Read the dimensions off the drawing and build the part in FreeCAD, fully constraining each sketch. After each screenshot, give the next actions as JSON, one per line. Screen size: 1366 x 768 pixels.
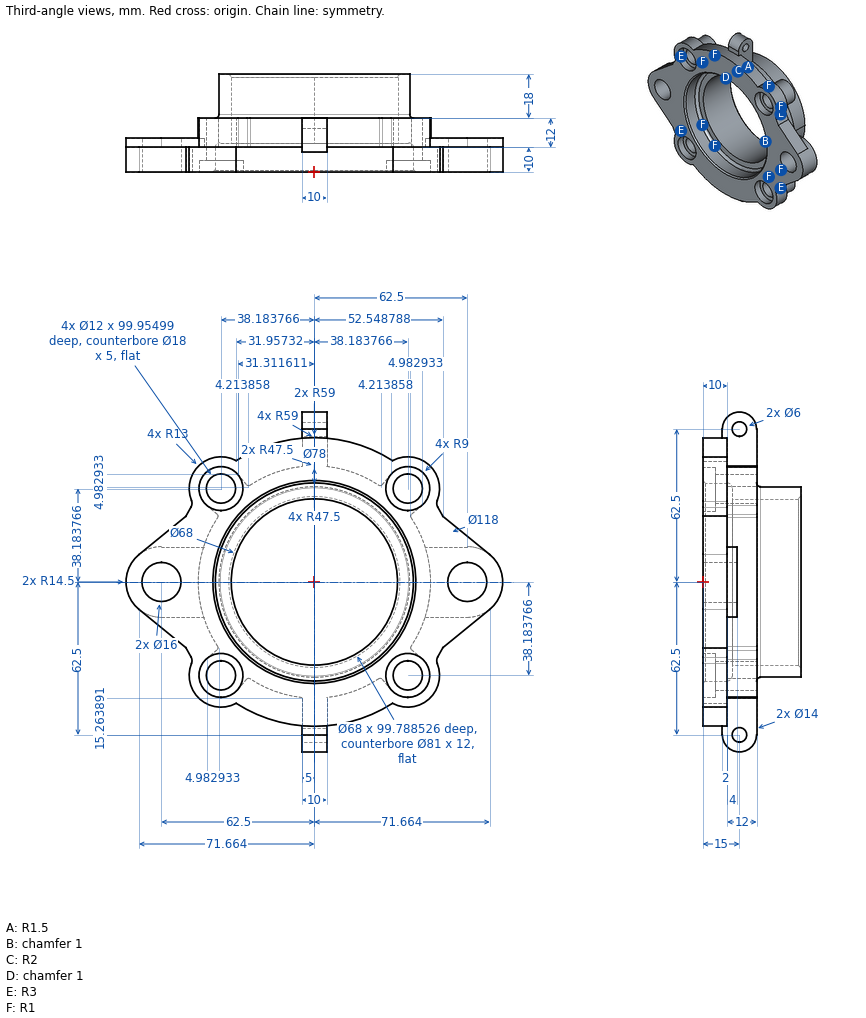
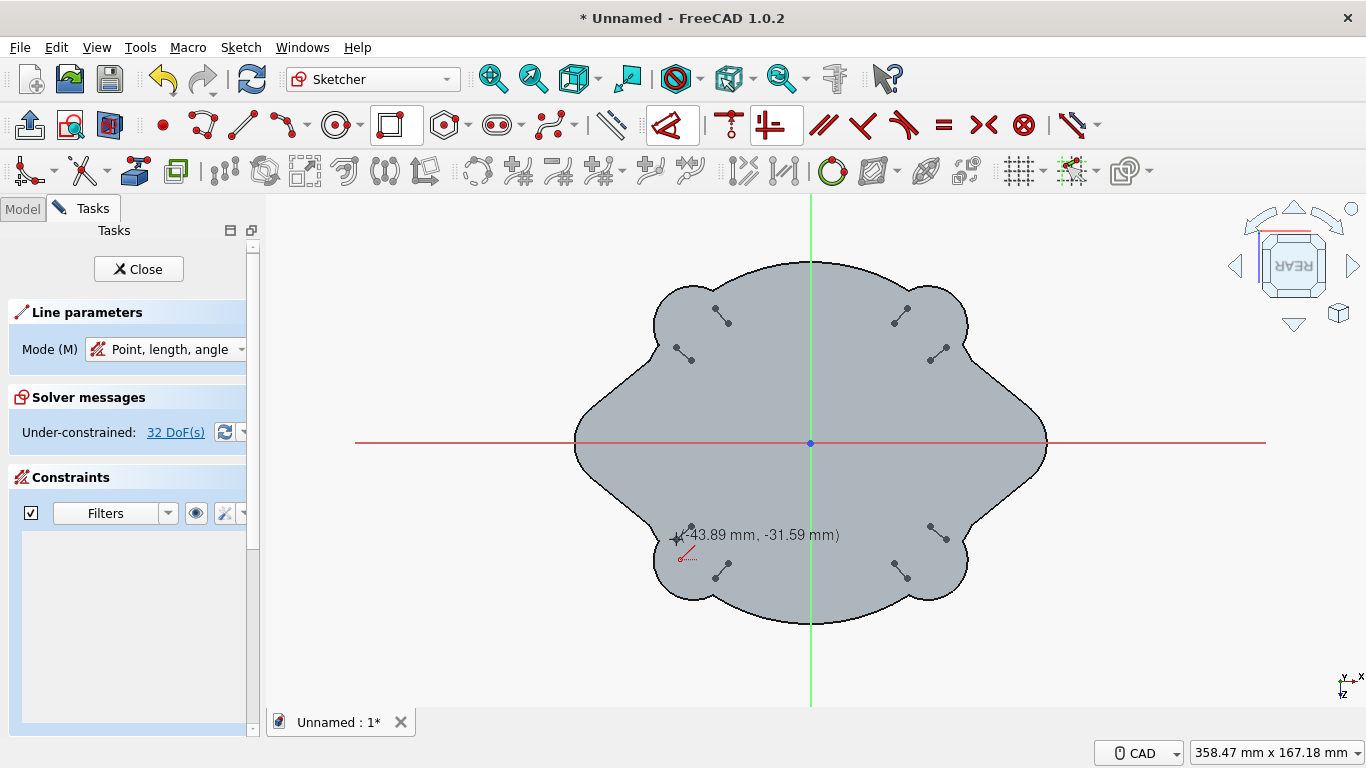
{"action": "left_click", "coordinate": [284, 126]}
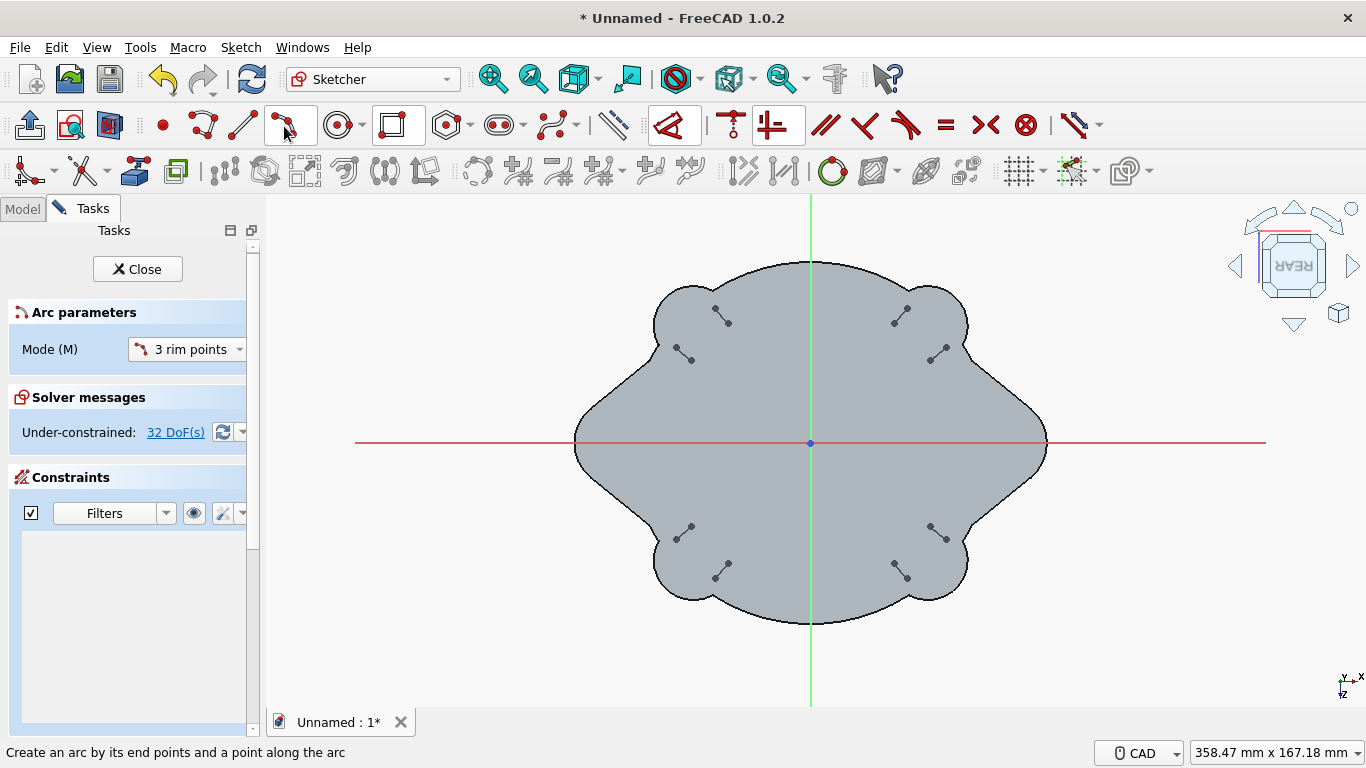
{"action": "scroll", "coordinate": [728, 563], "scroll_direction": "up", "scroll_amount": 3}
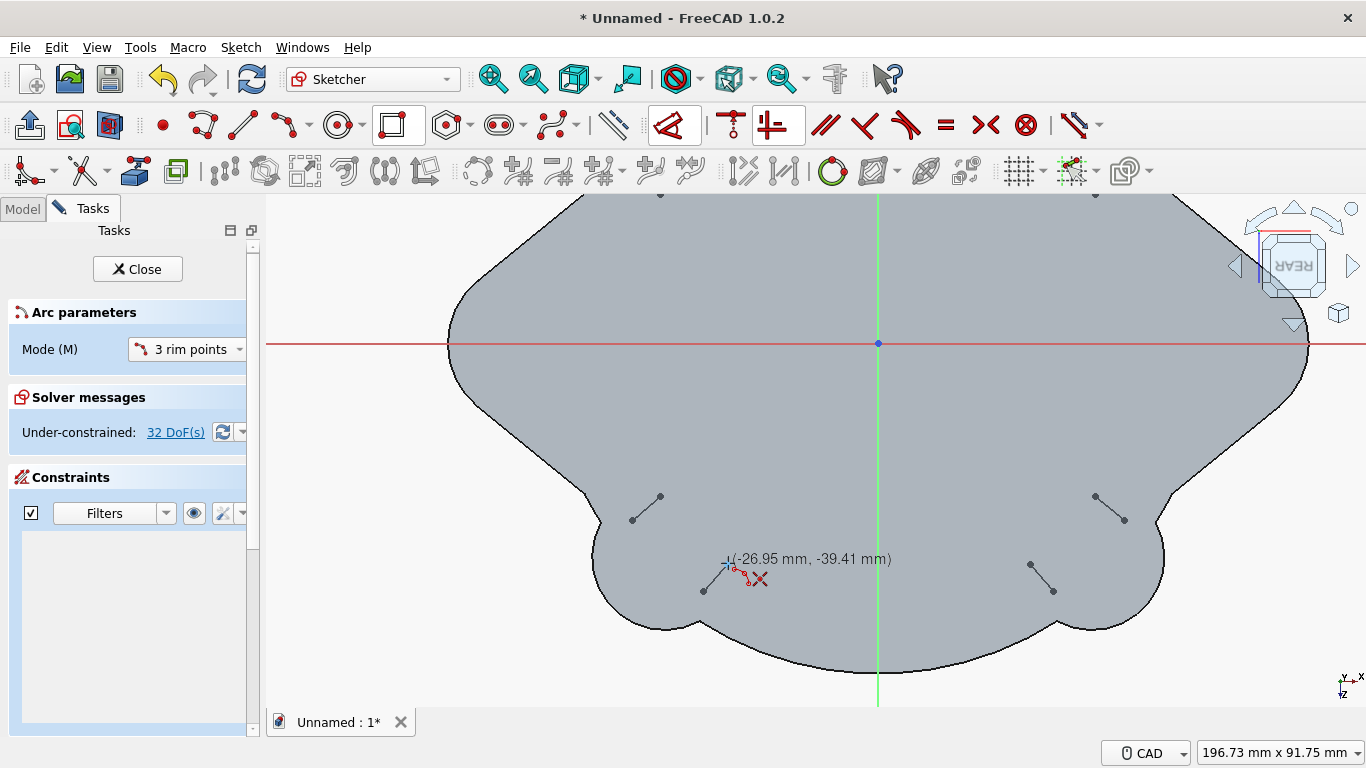
{"action": "left_click", "coordinate": [728, 564]}
{"action": "left_click", "coordinate": [1030, 564]}
{"action": "left_click", "coordinate": [846, 608]}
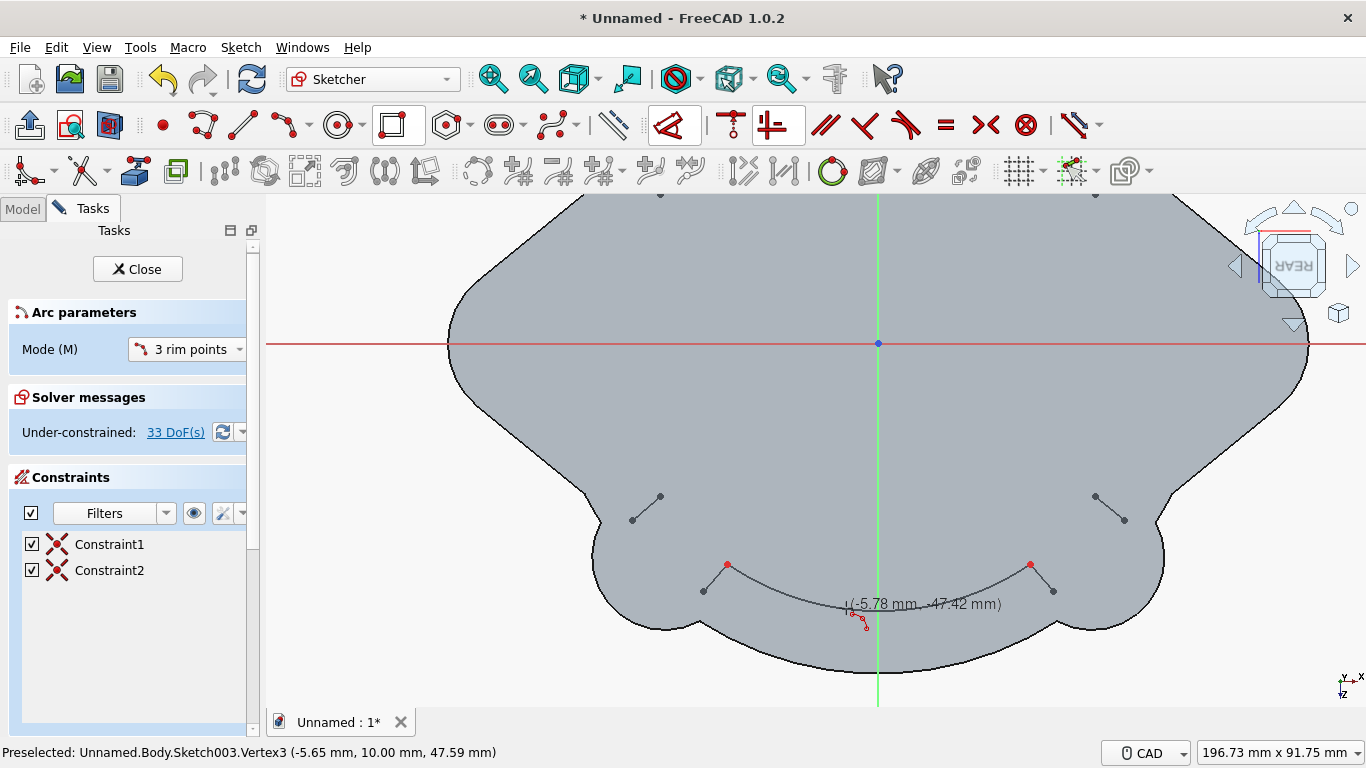
{"action": "left_click", "coordinate": [1054, 592]}
{"action": "left_click", "coordinate": [1125, 520]}
{"action": "left_click", "coordinate": [1127, 593]}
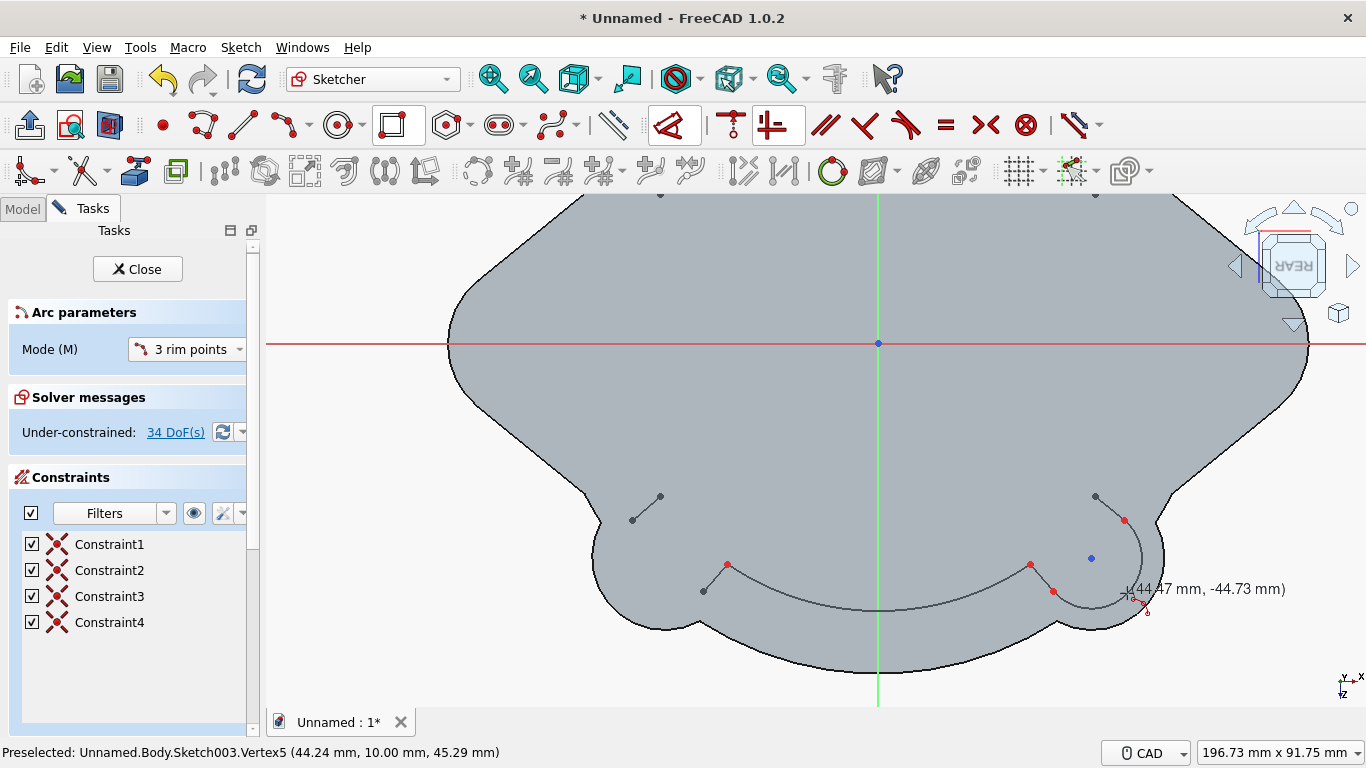
{"action": "left_click", "coordinate": [1096, 497]}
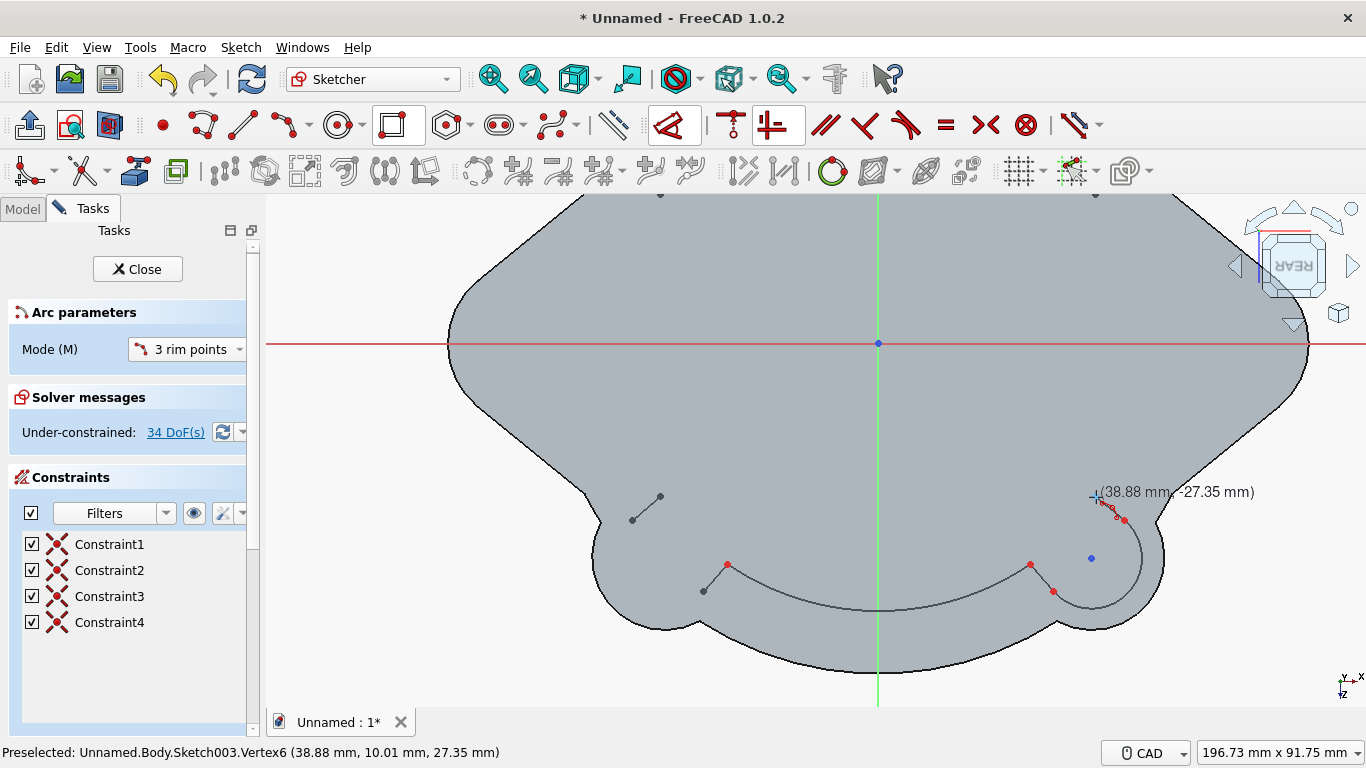
{"action": "scroll", "coordinate": [481, 667], "scroll_direction": "down", "scroll_amount": 2}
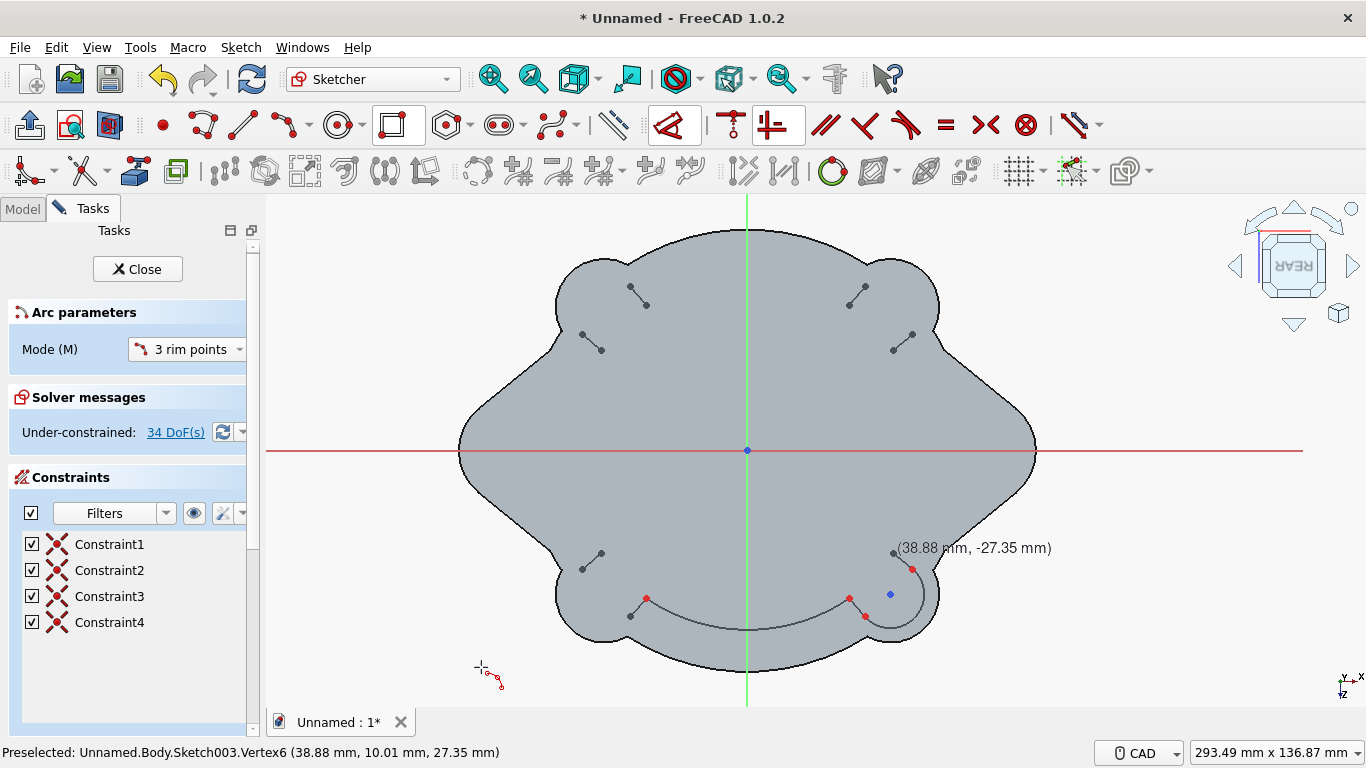
{"action": "scroll", "coordinate": [894, 349], "scroll_direction": "up", "scroll_amount": 2}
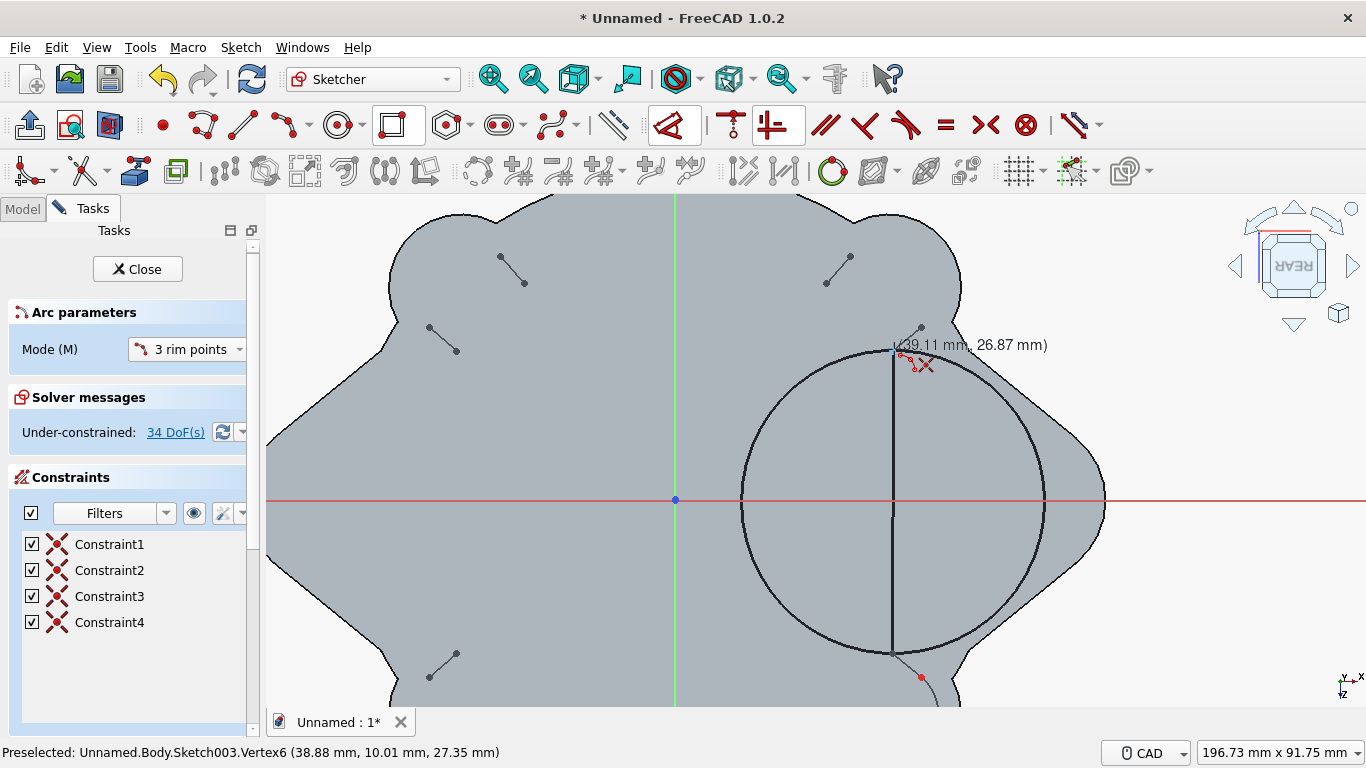
{"action": "left_click", "coordinate": [892, 351]}
{"action": "left_click", "coordinate": [939, 533]}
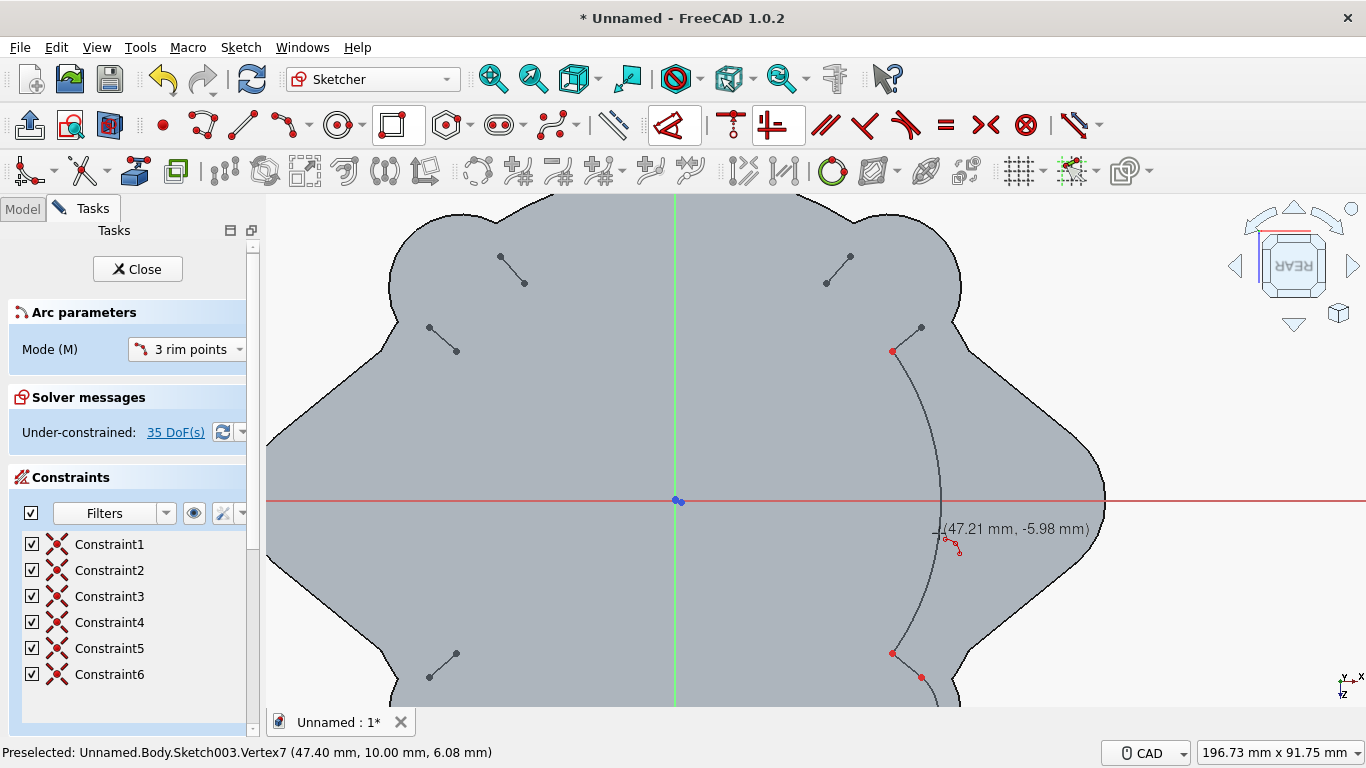
{"action": "left_click", "coordinate": [922, 327]}
{"action": "left_click", "coordinate": [851, 256]}
{"action": "left_click", "coordinate": [924, 251]}